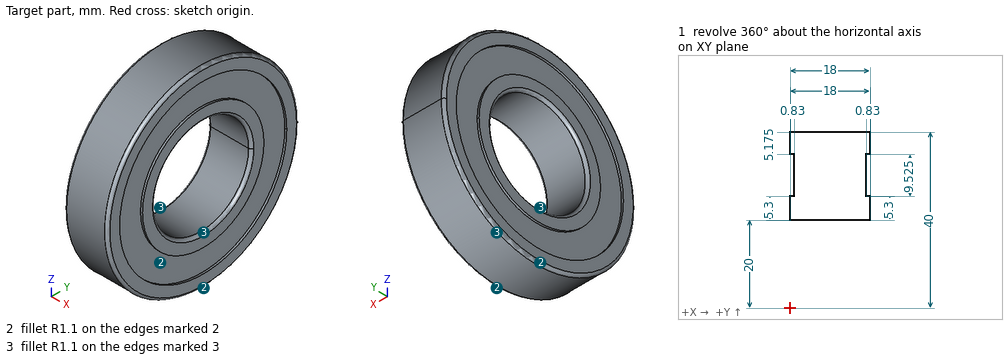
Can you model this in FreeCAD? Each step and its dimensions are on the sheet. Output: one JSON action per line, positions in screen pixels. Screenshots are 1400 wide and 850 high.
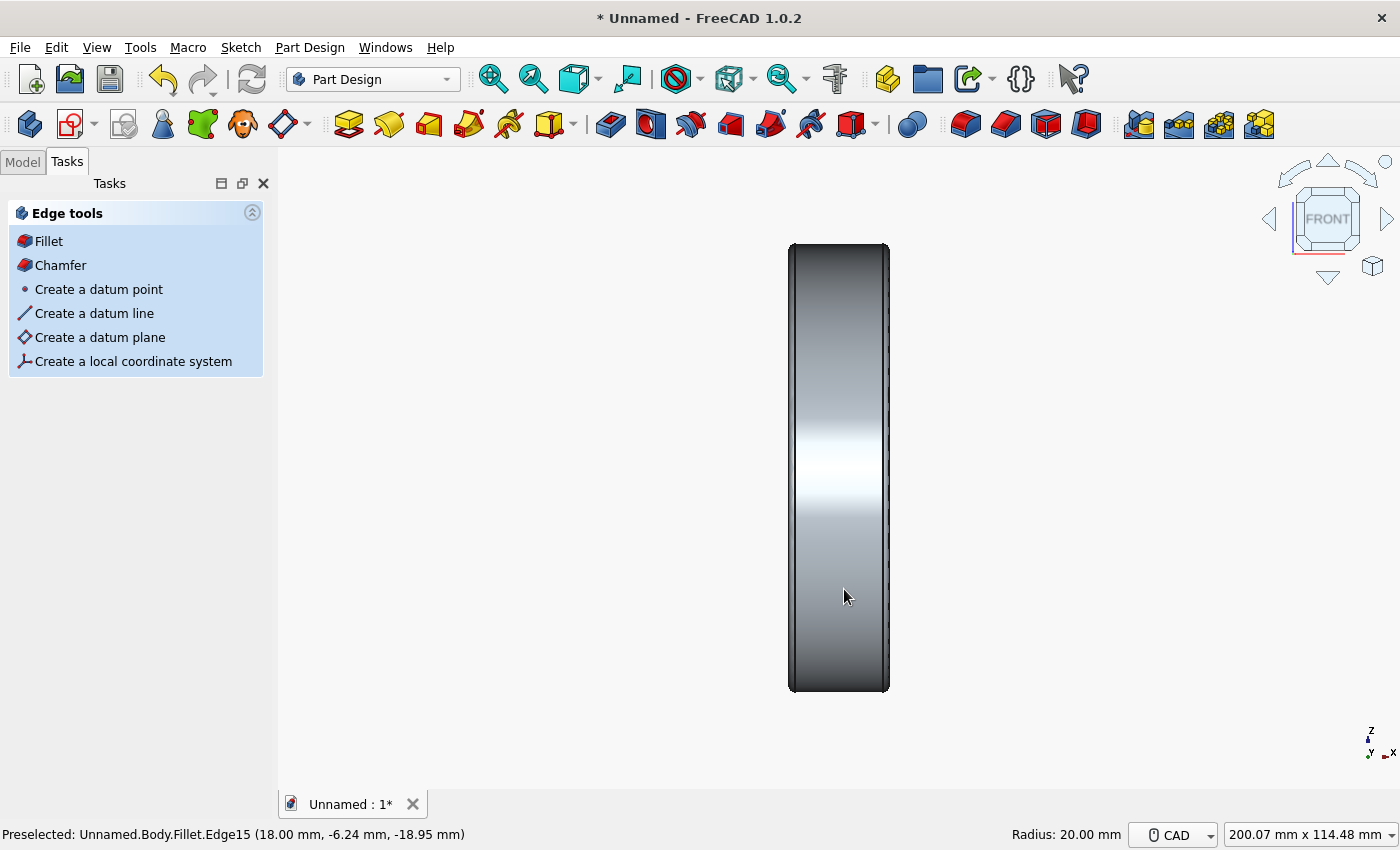
{"action": "key", "text": "3"}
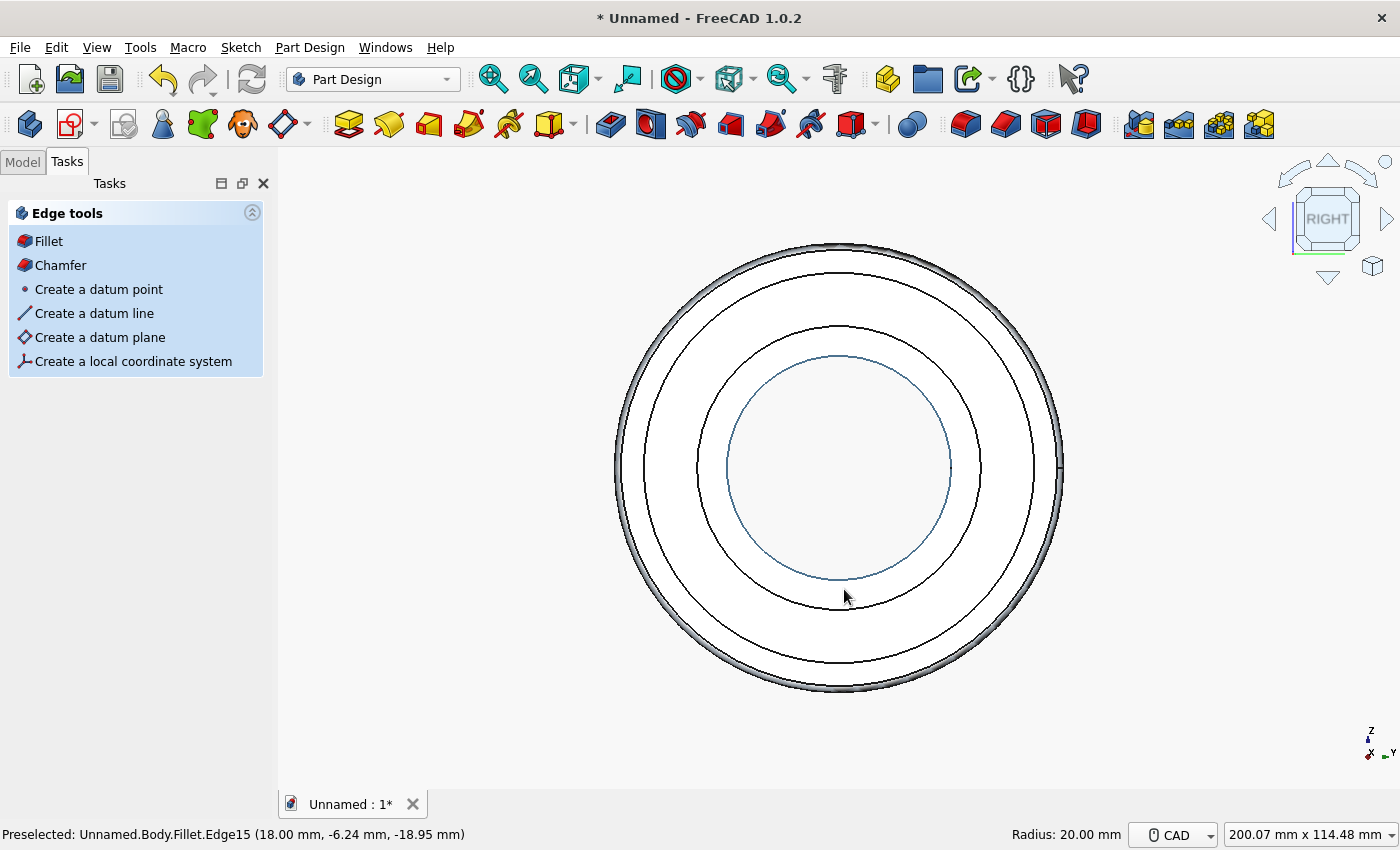
{"action": "key", "text": "5"}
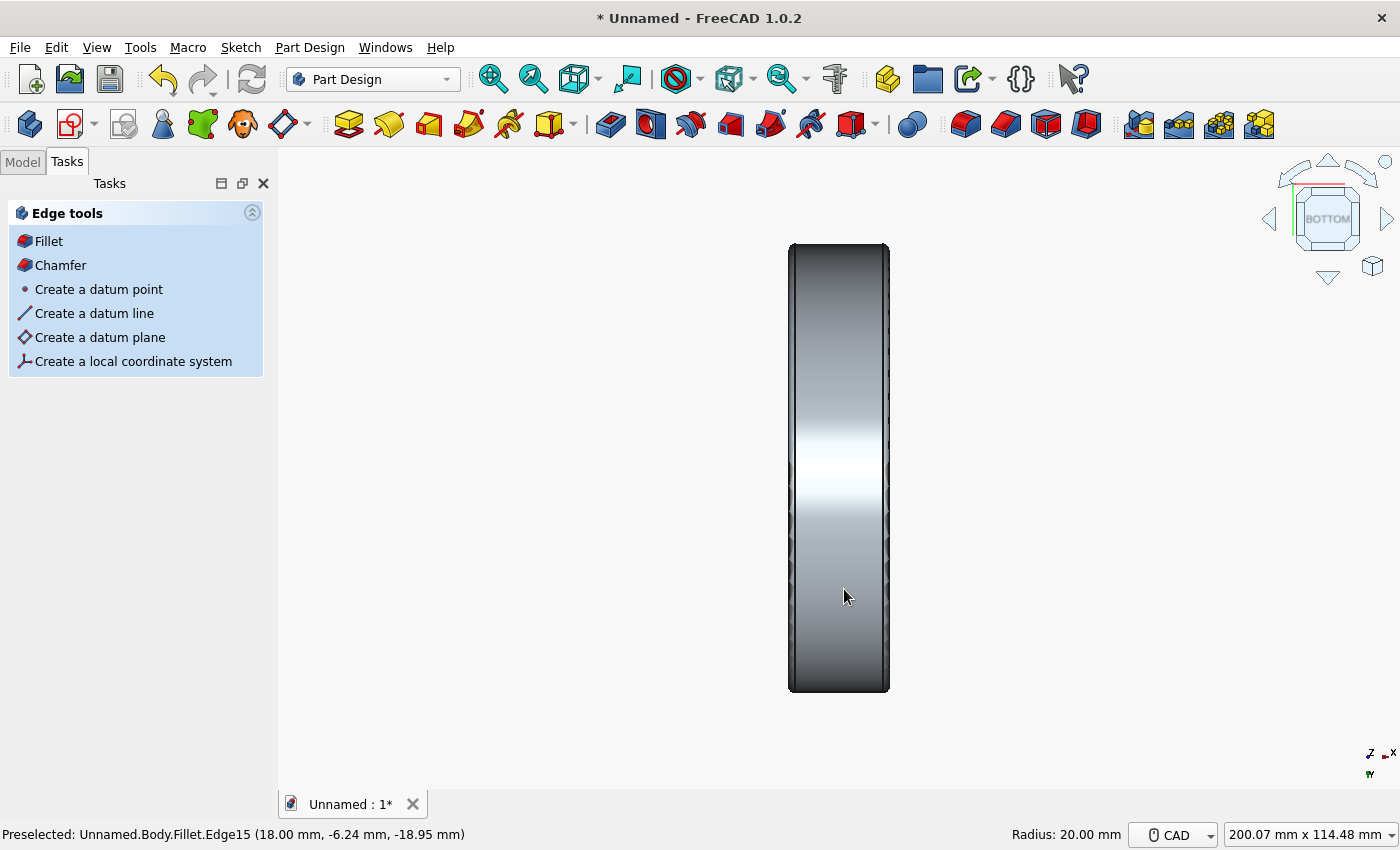
{"action": "key", "text": "4"}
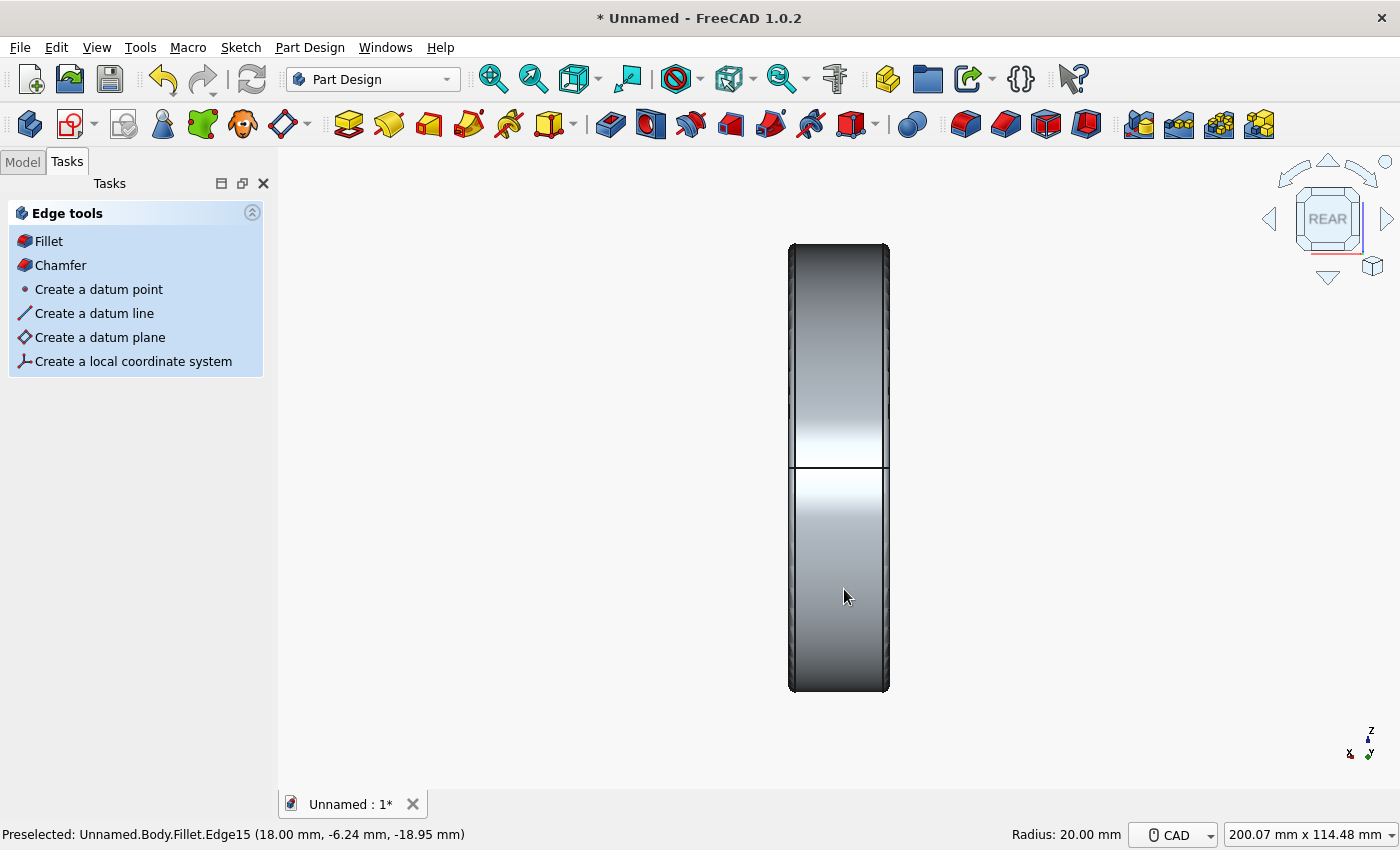
{"action": "key", "text": "6"}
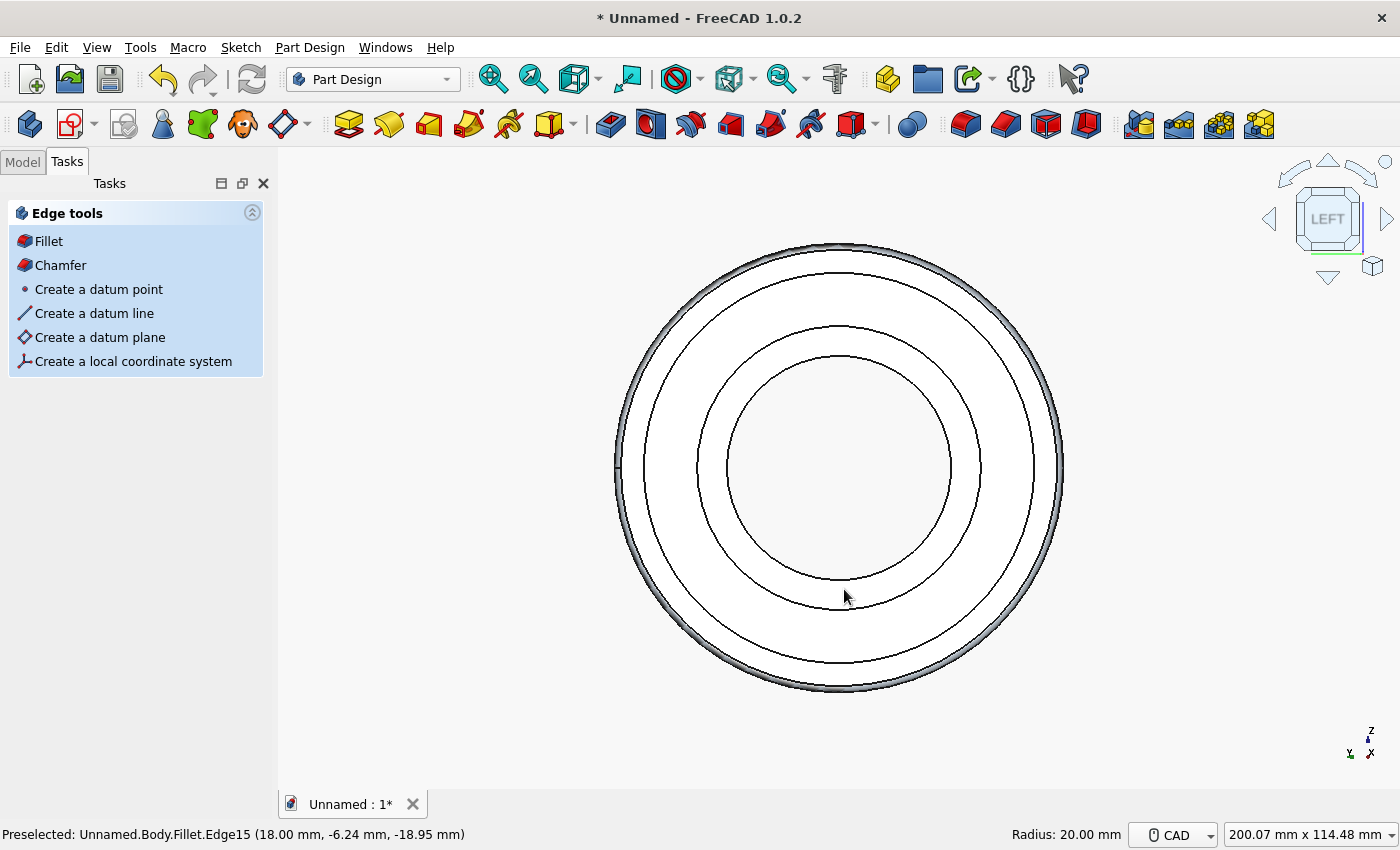
{"action": "left_click", "coordinate": [951, 467], "text": "ctrl"}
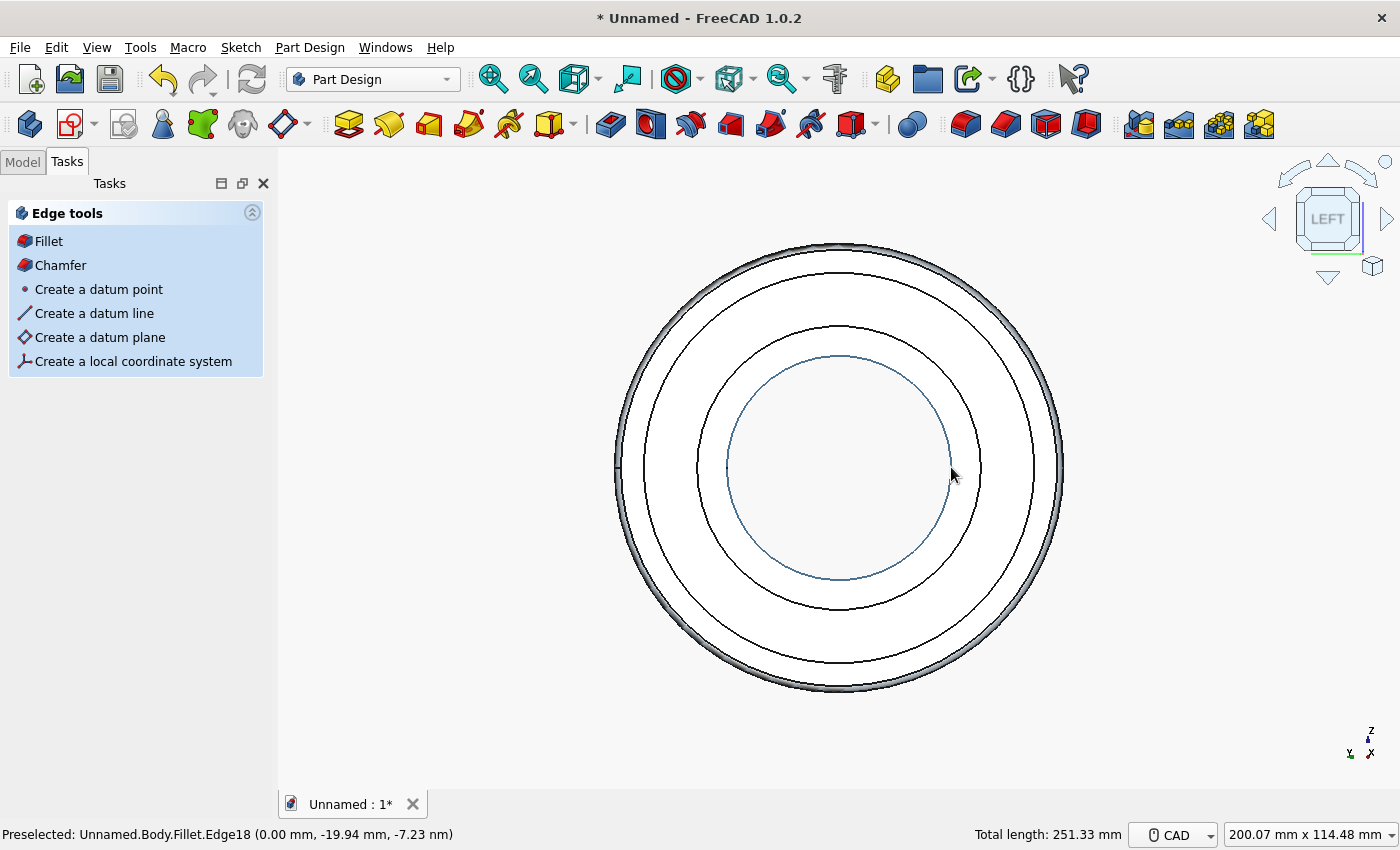
{"action": "left_click", "coordinate": [966, 124]}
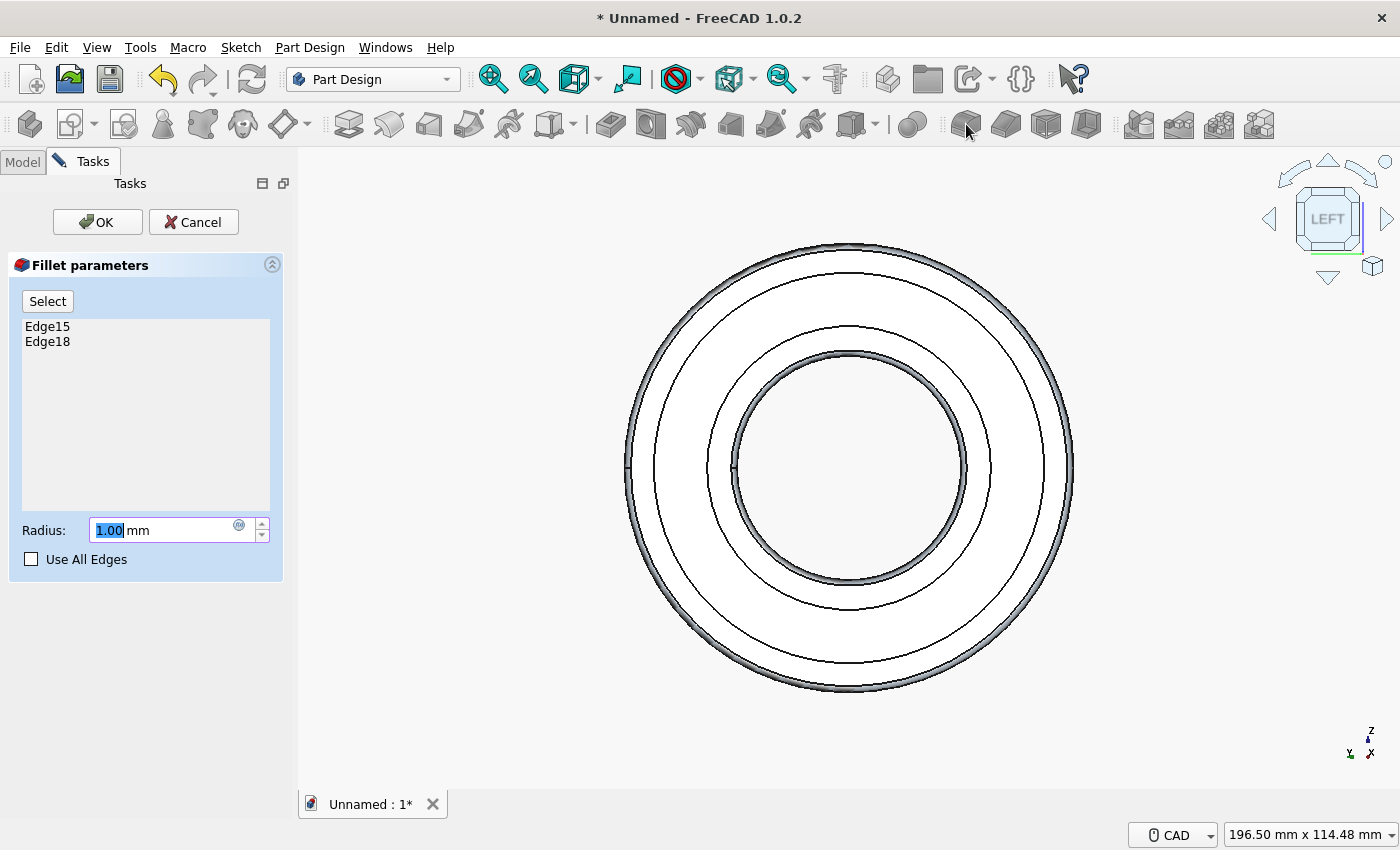
{"action": "type", "text": "1.1"}
{"action": "key", "text": "Tab"}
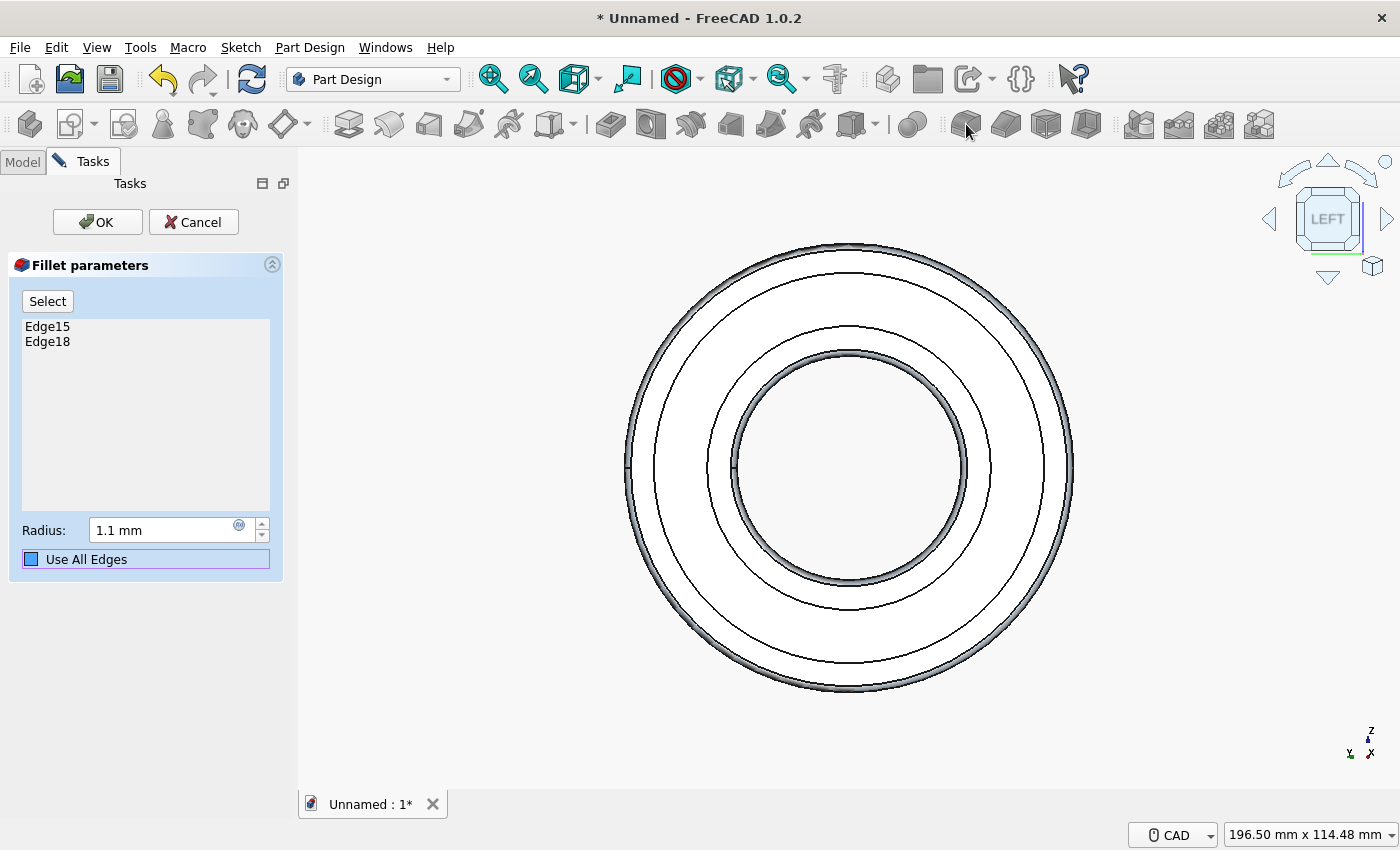
{"action": "left_click", "coordinate": [98, 222]}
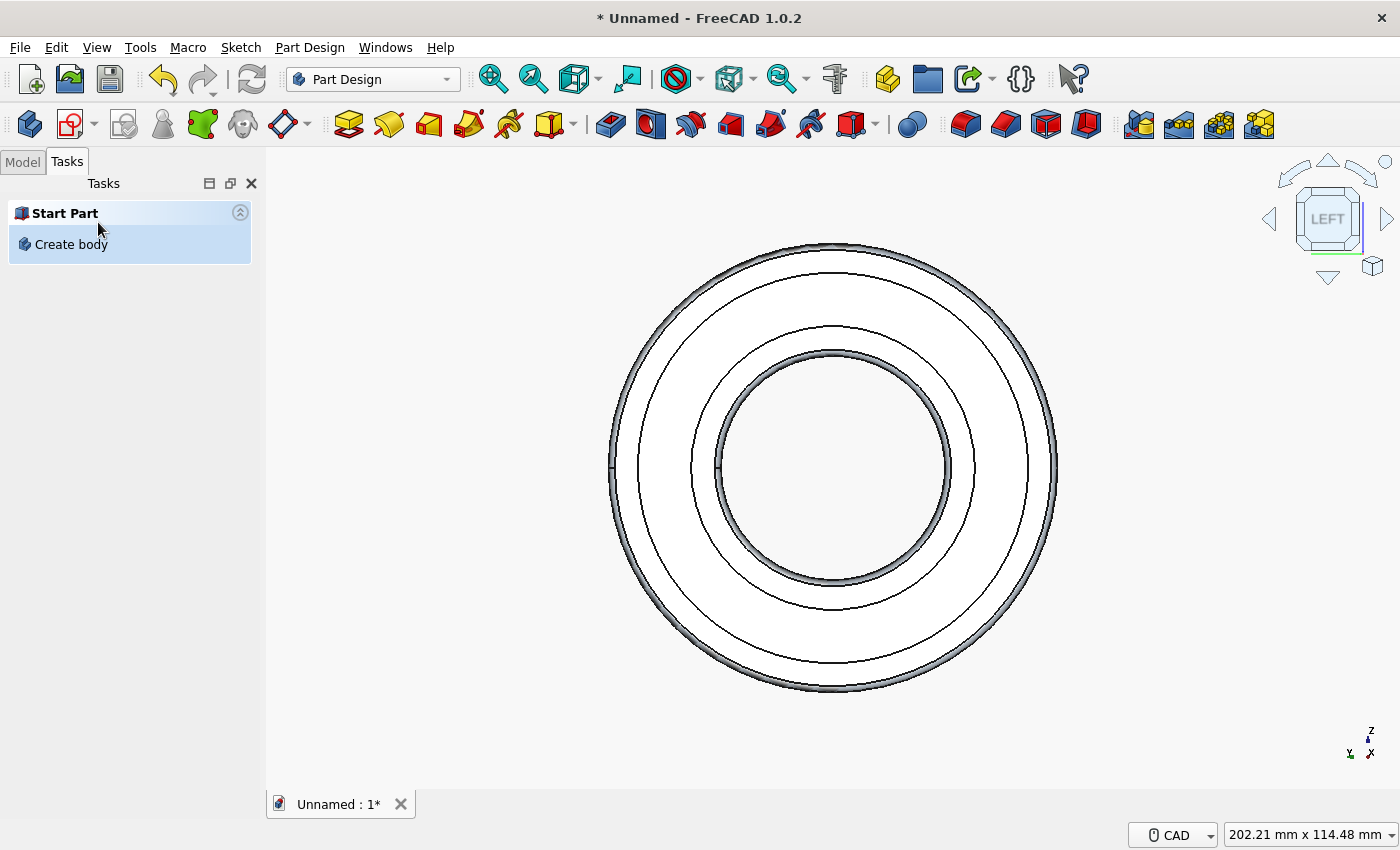
{"action": "key", "text": "0"}